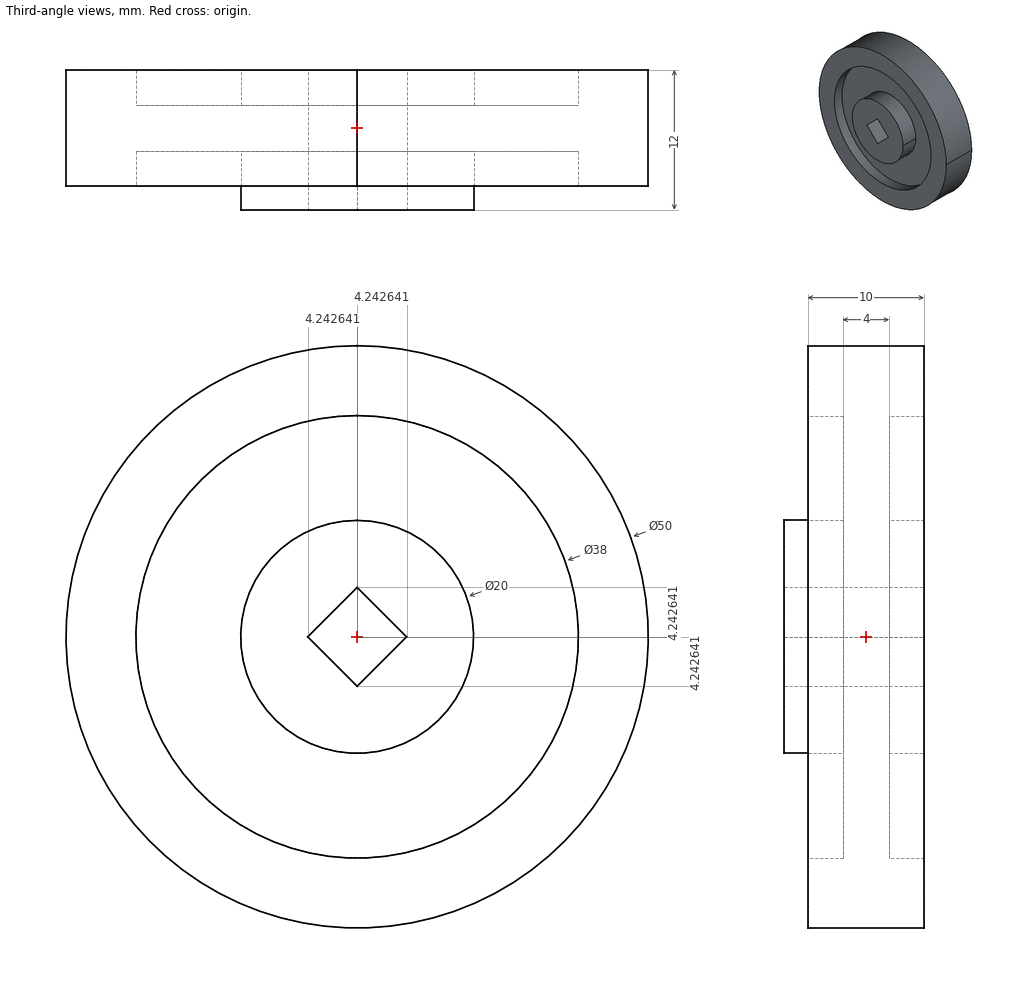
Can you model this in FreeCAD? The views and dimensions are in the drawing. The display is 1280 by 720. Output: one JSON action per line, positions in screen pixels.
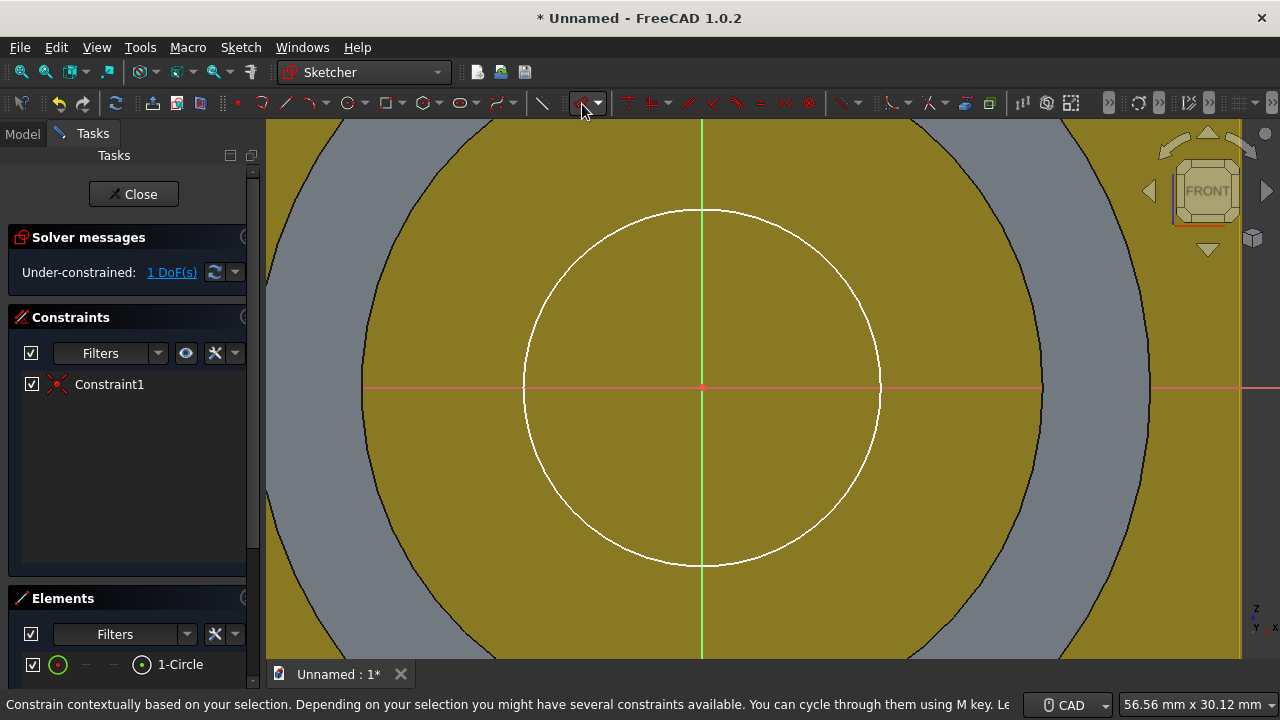
{"action": "left_click", "coordinate": [828, 261]}
{"action": "left_click", "coordinate": [851, 238]}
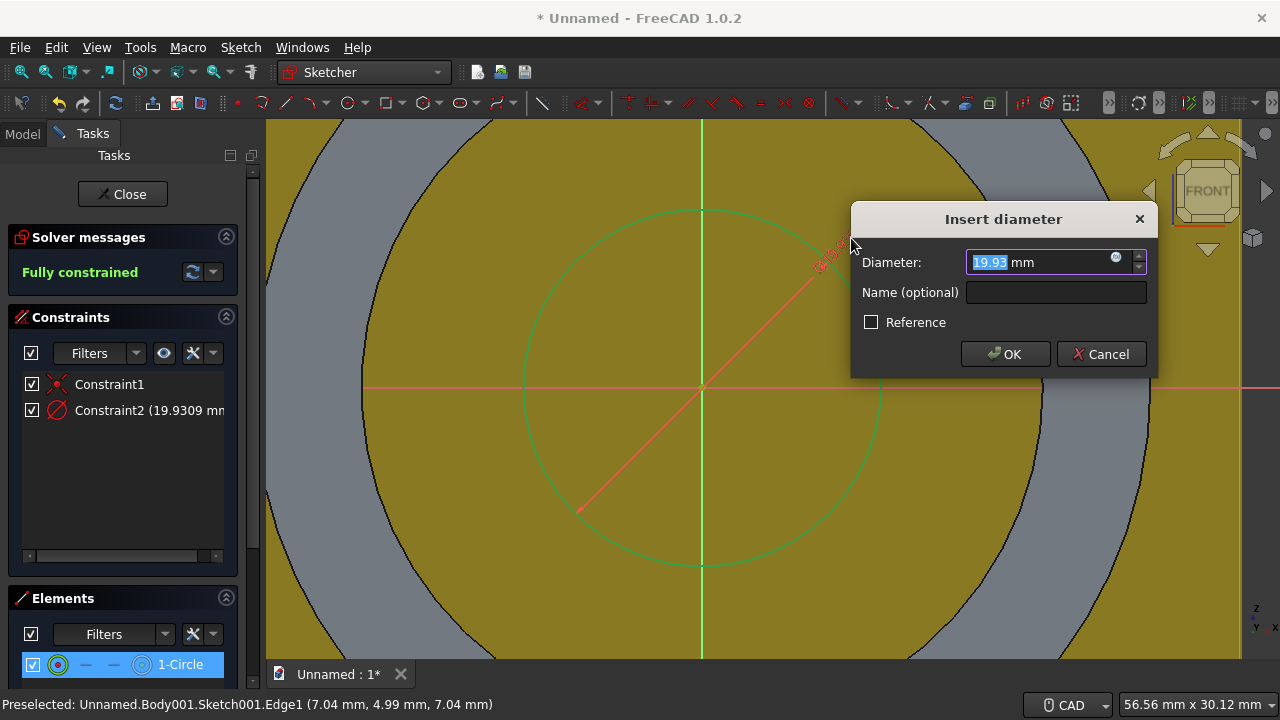
{"action": "type", "text": "20"}
{"action": "key", "text": "Return"}
{"action": "key", "text": "Escape"}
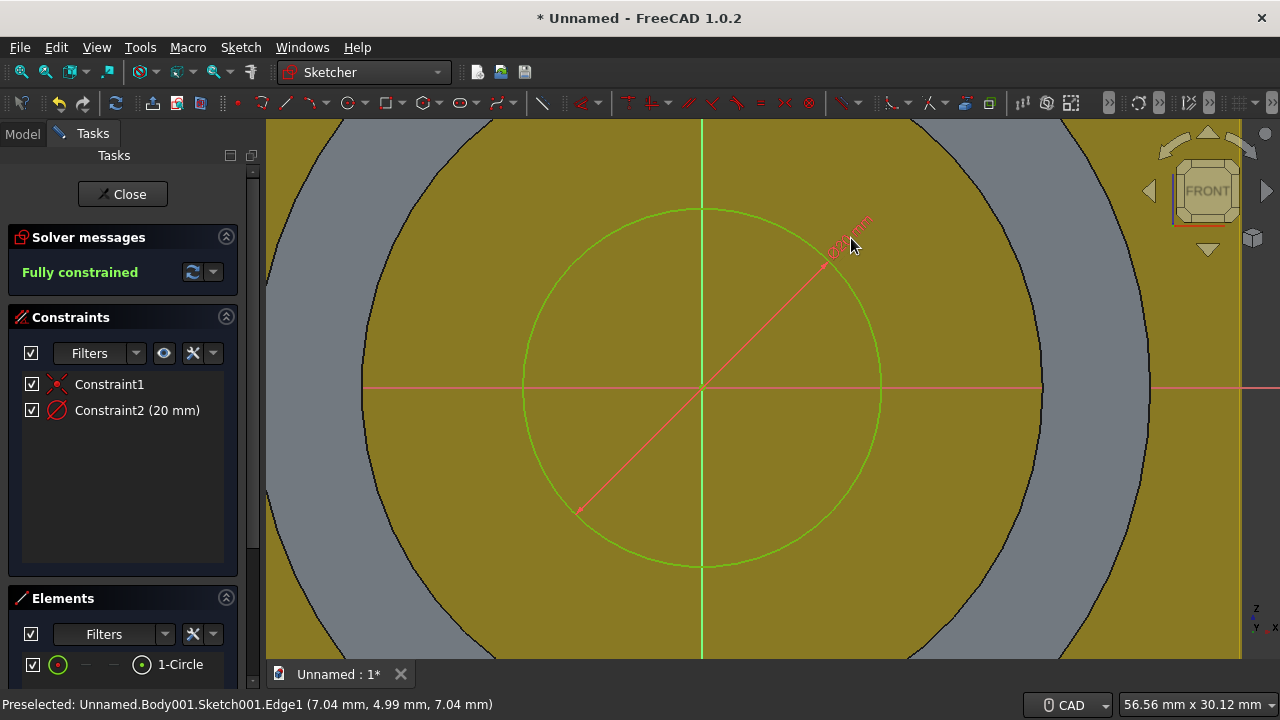
{"action": "left_click", "coordinate": [123, 194]}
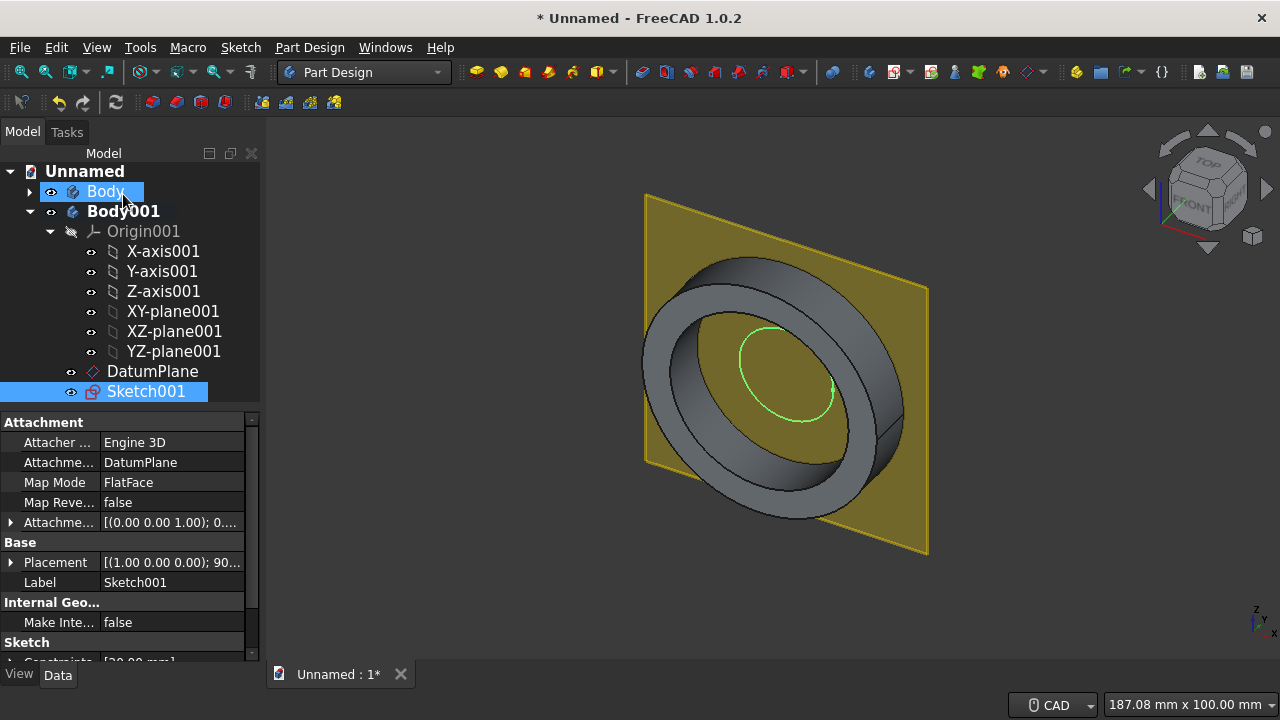
{"action": "left_click", "coordinate": [478, 72]}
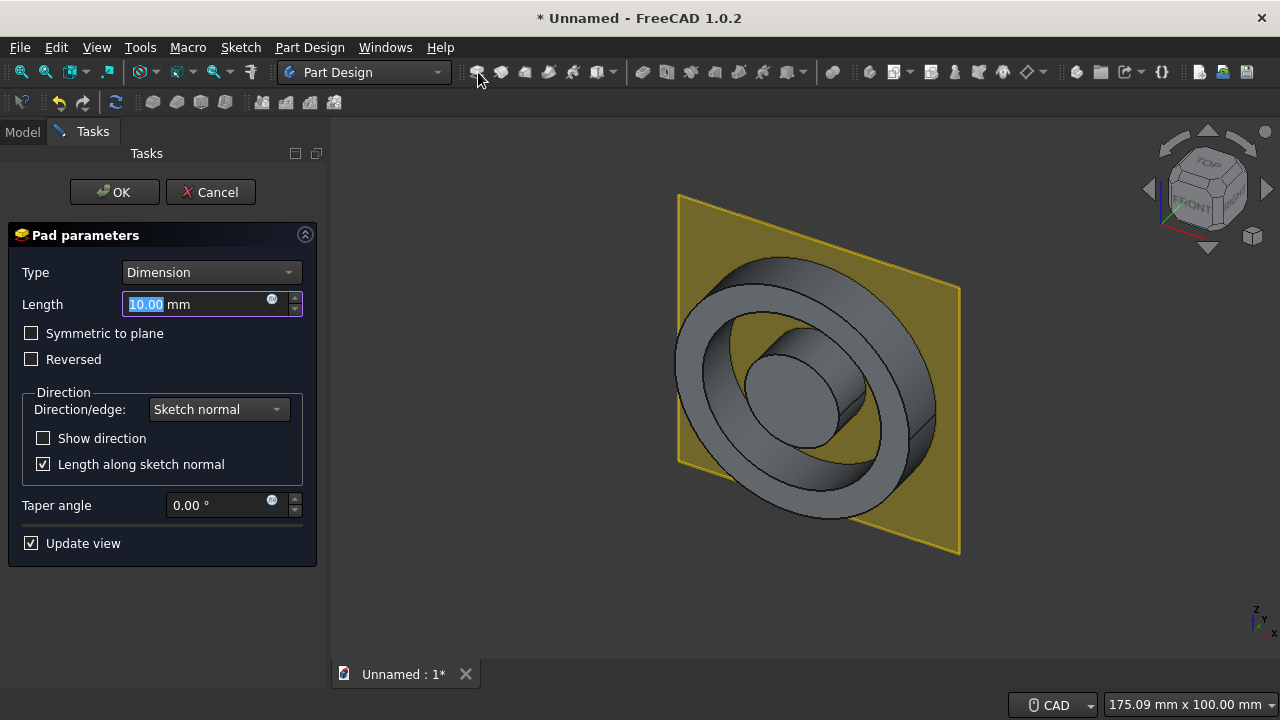
{"action": "type", "text": "12"}
{"action": "key", "text": "Tab"}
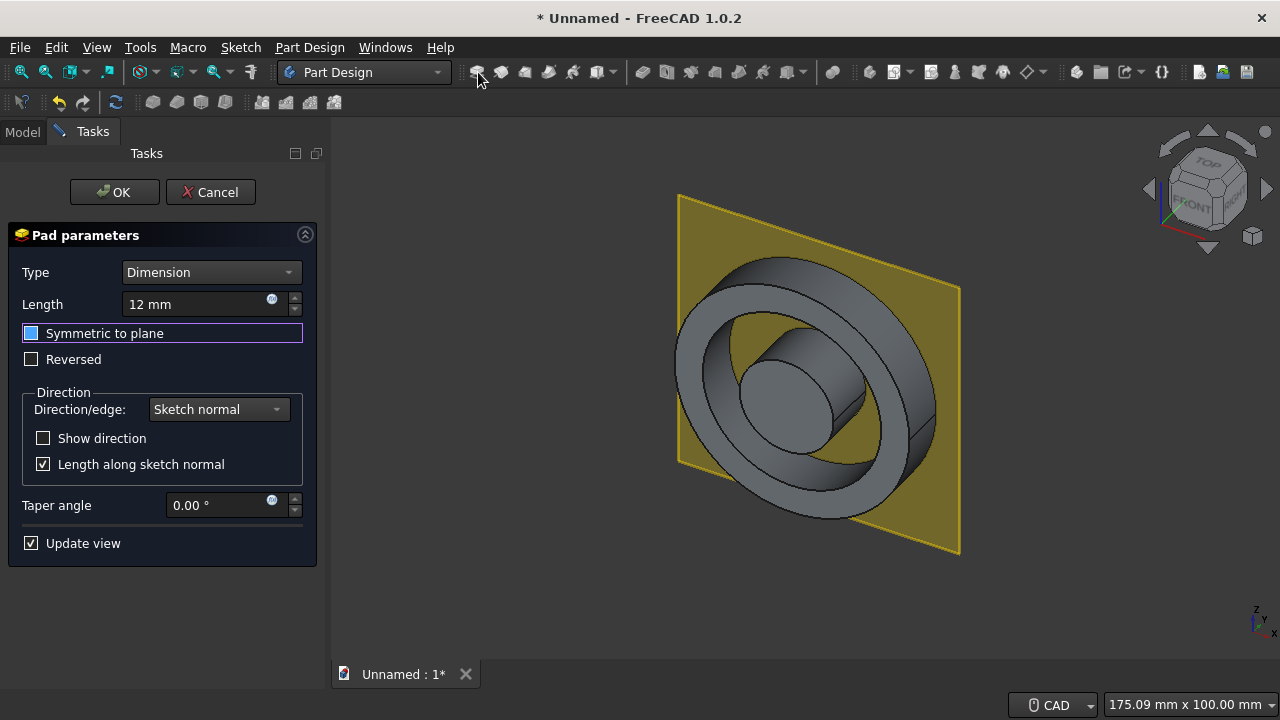
{"action": "left_click", "coordinate": [115, 192]}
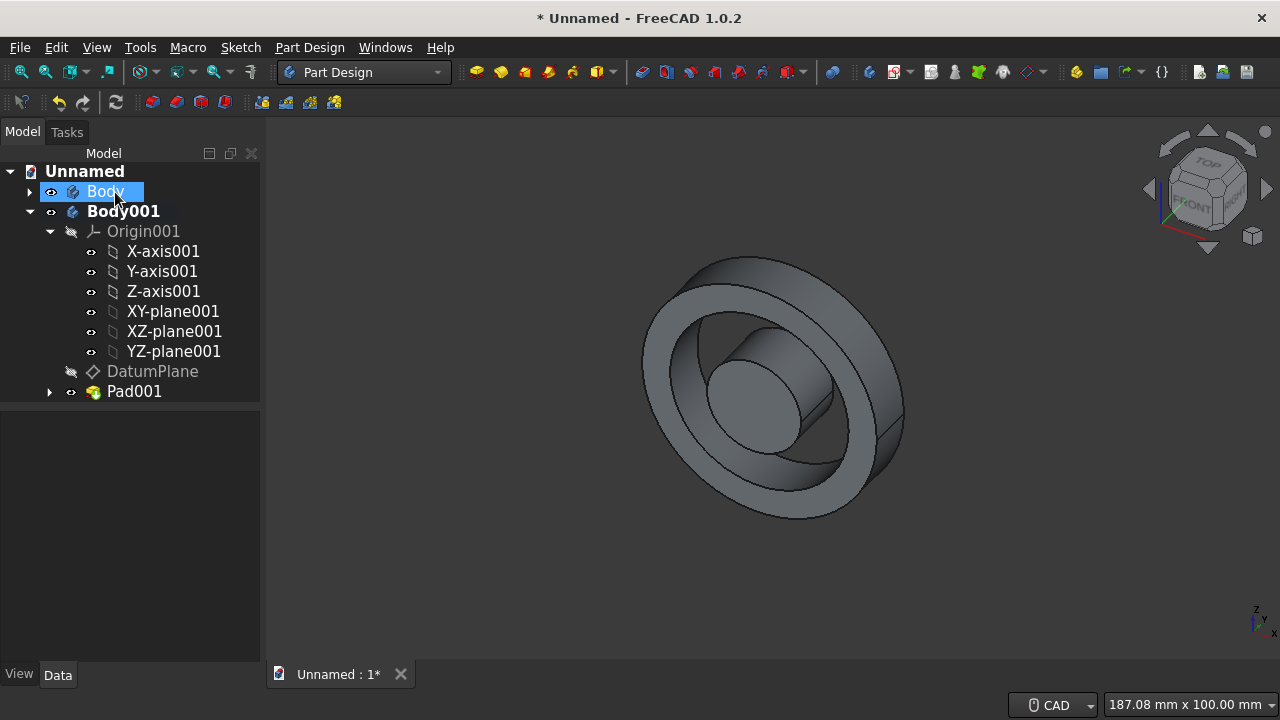
{"action": "left_click", "coordinate": [22, 72]}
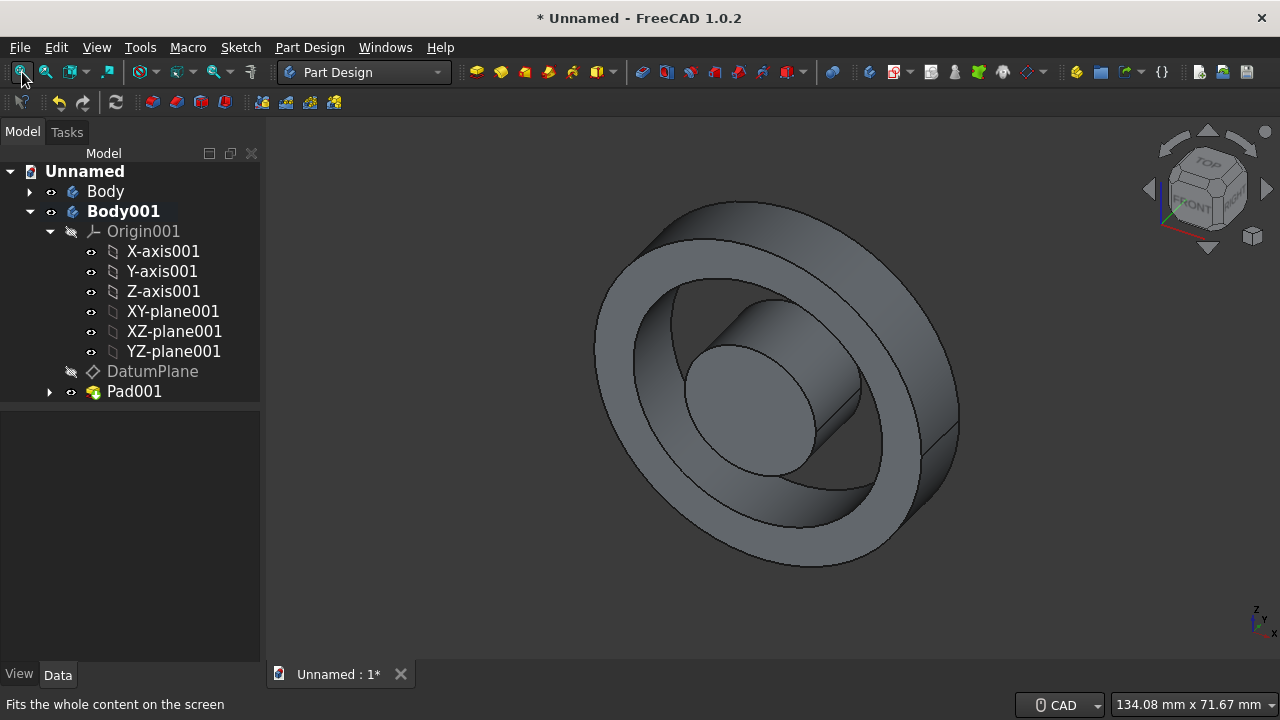
{"action": "double_click", "coordinate": [96, 192]}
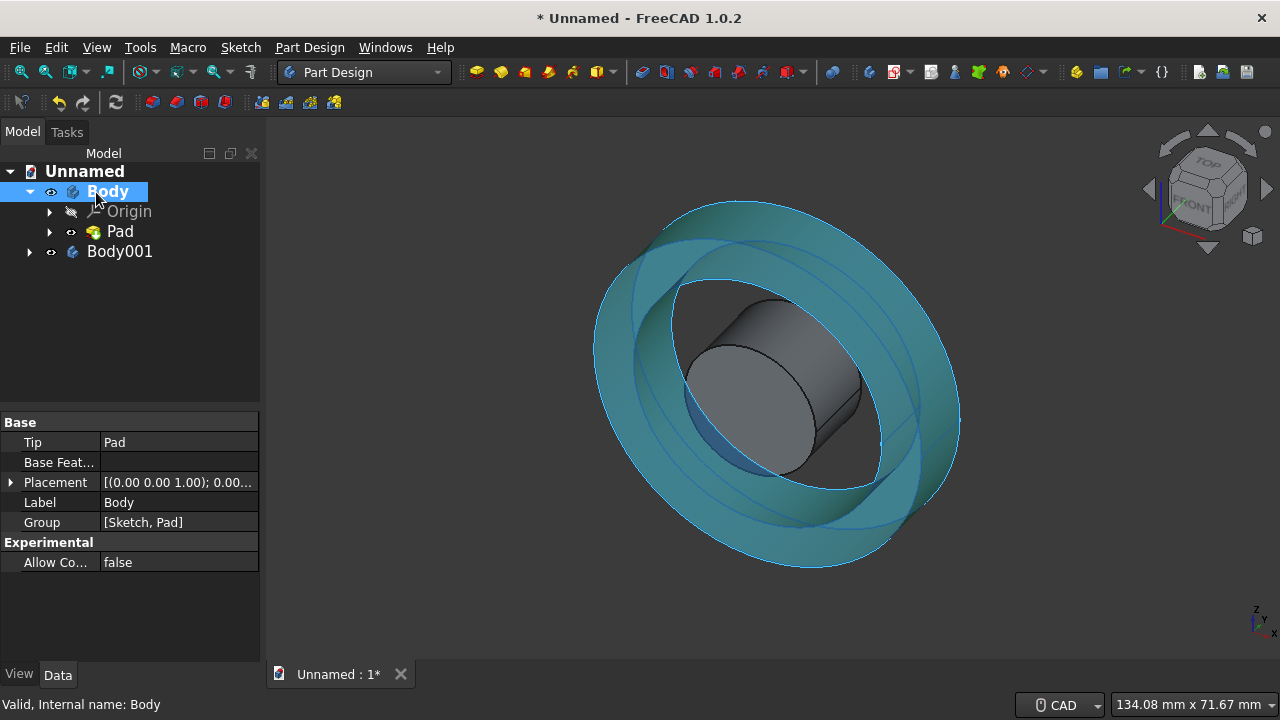
{"action": "left_click", "coordinate": [96, 192]}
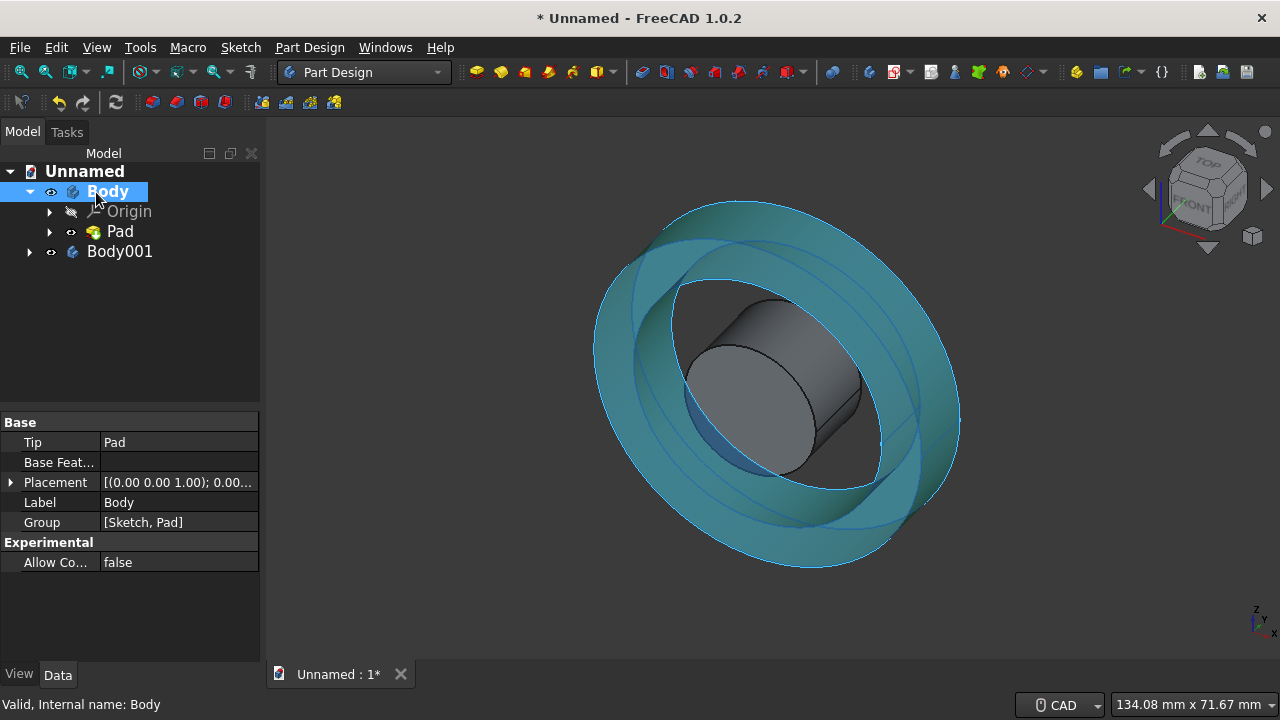
{"action": "left_click", "coordinate": [146, 562]}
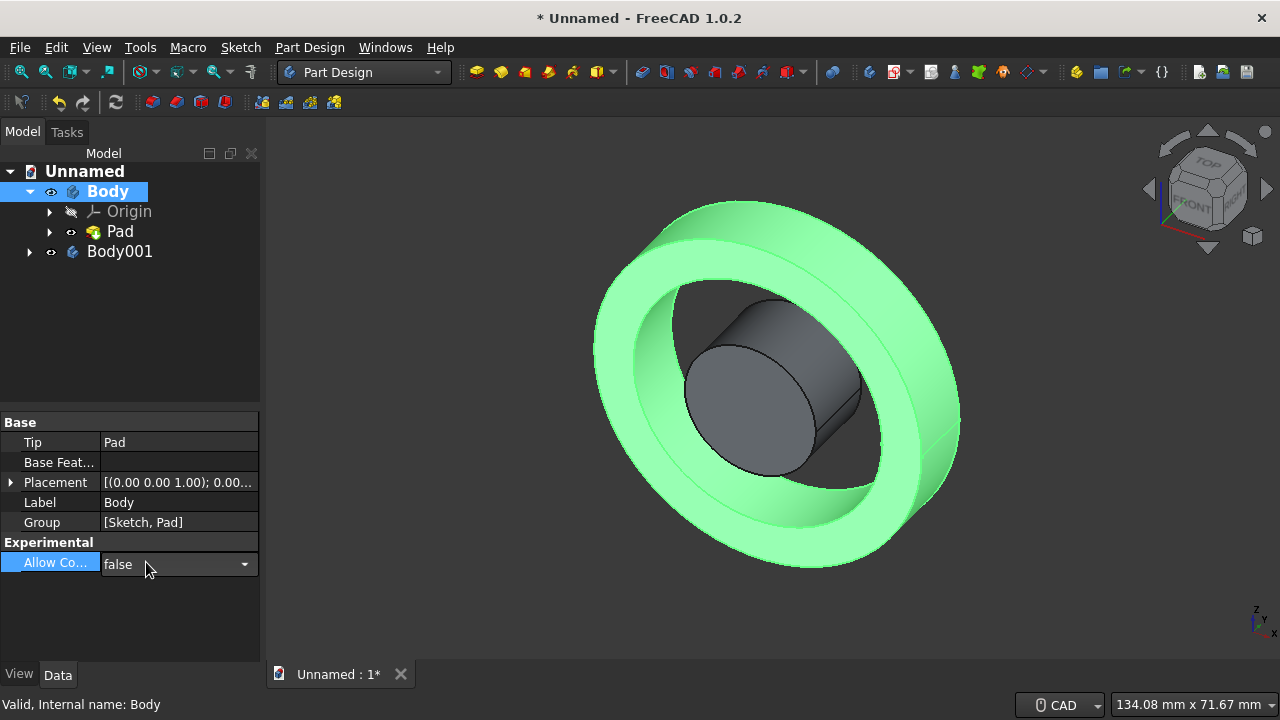
{"action": "left_click", "coordinate": [146, 562]}